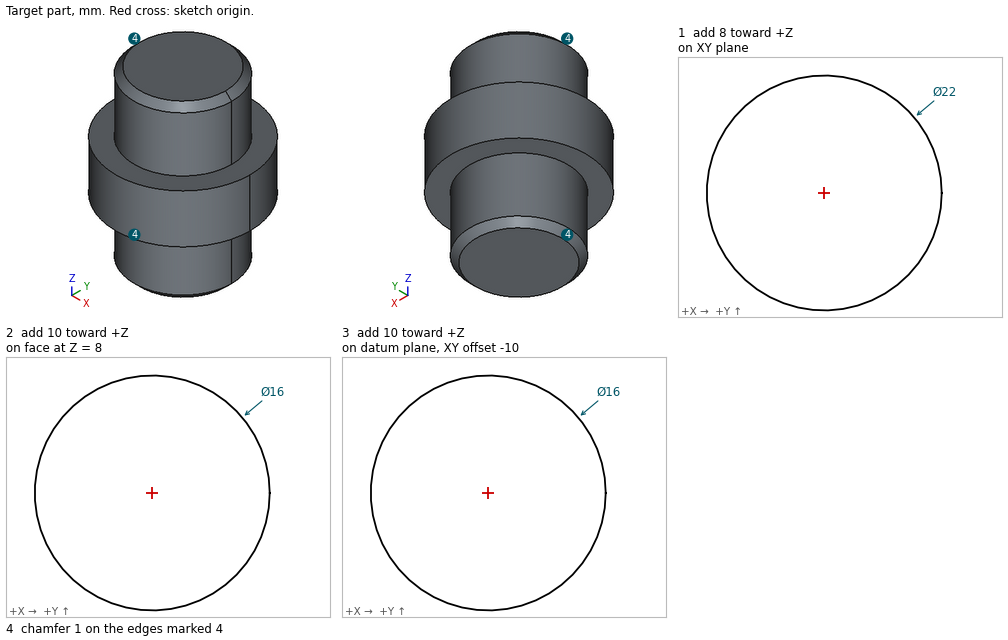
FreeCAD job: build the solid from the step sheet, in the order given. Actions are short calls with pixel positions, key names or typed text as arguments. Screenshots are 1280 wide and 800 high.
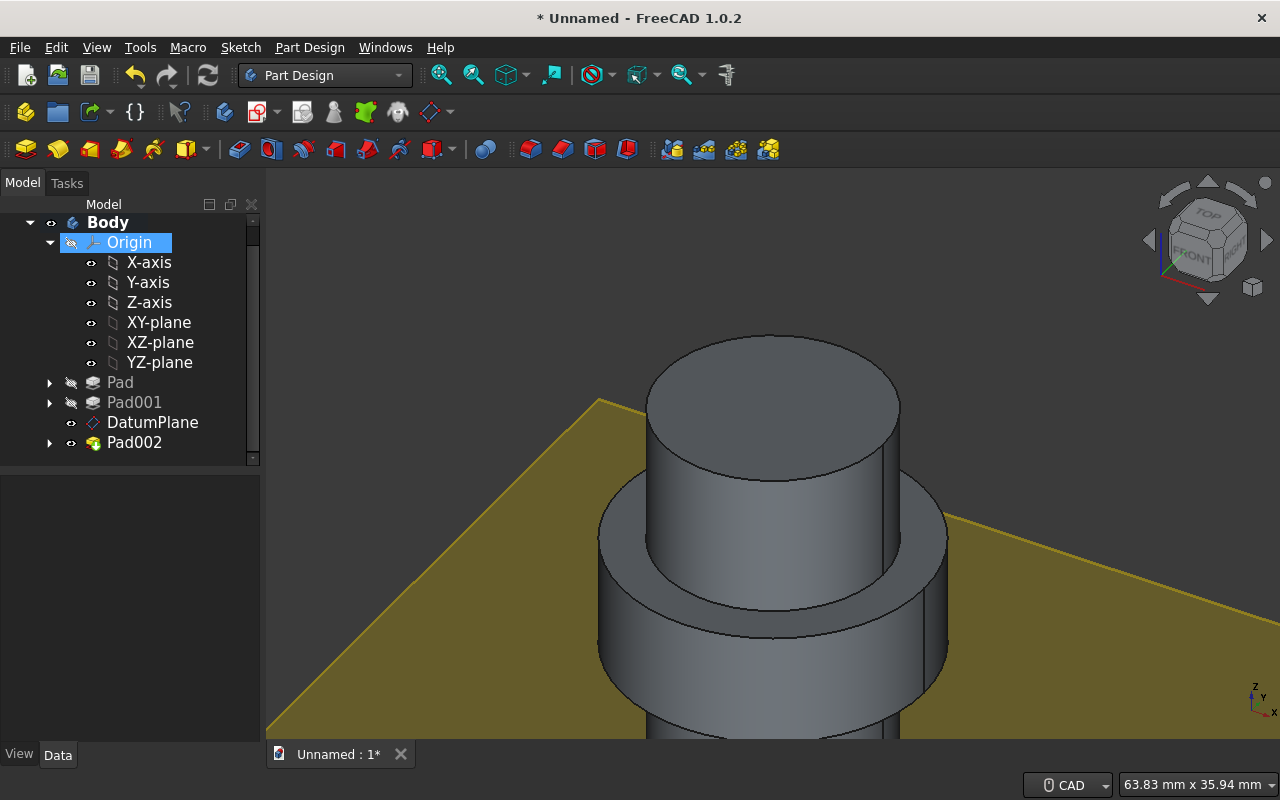
click(116, 423)
key(space)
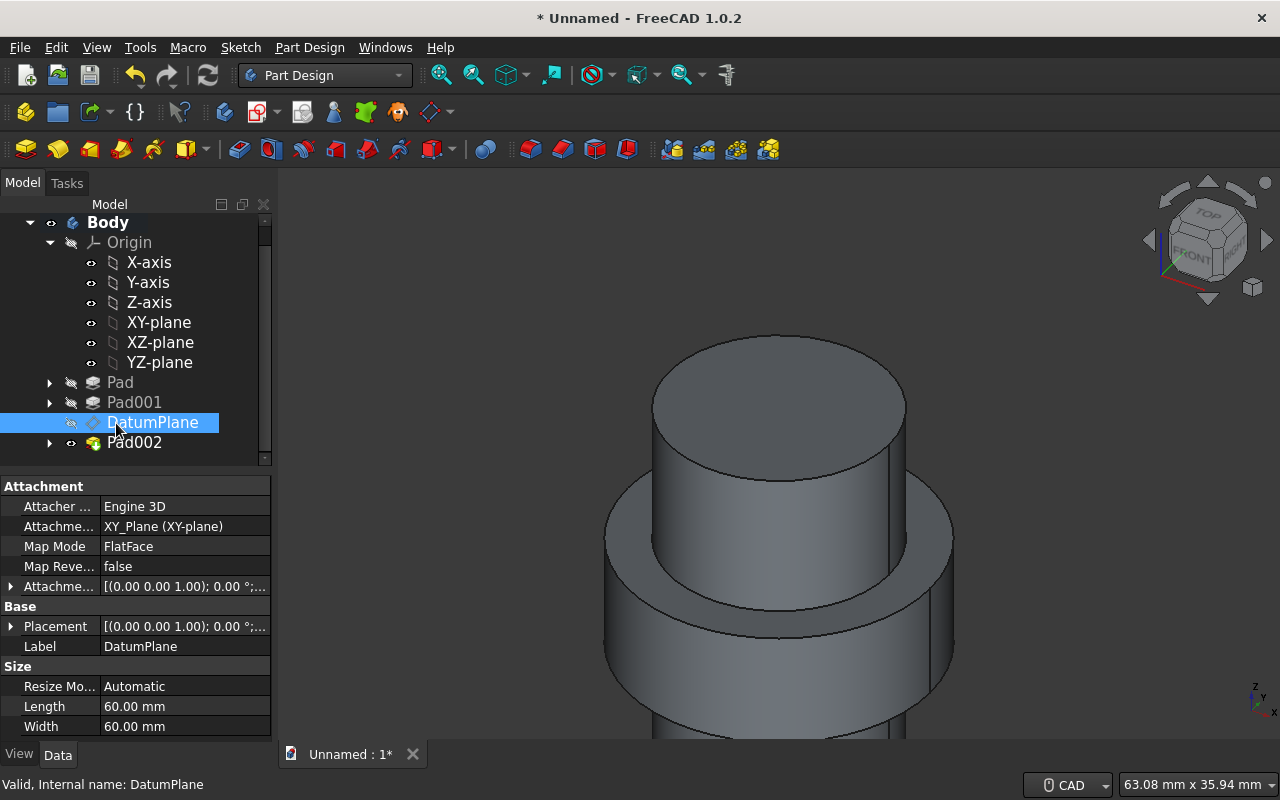
click(442, 76)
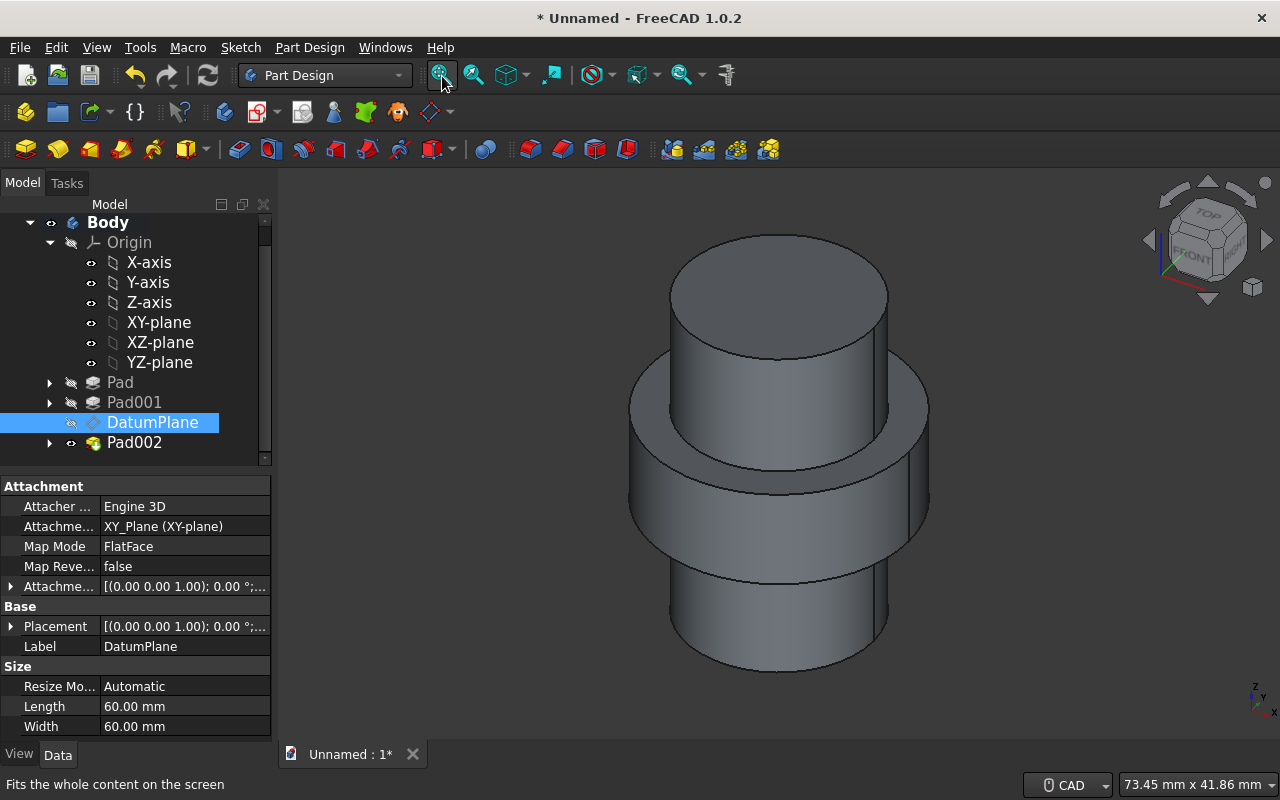
click(698, 651)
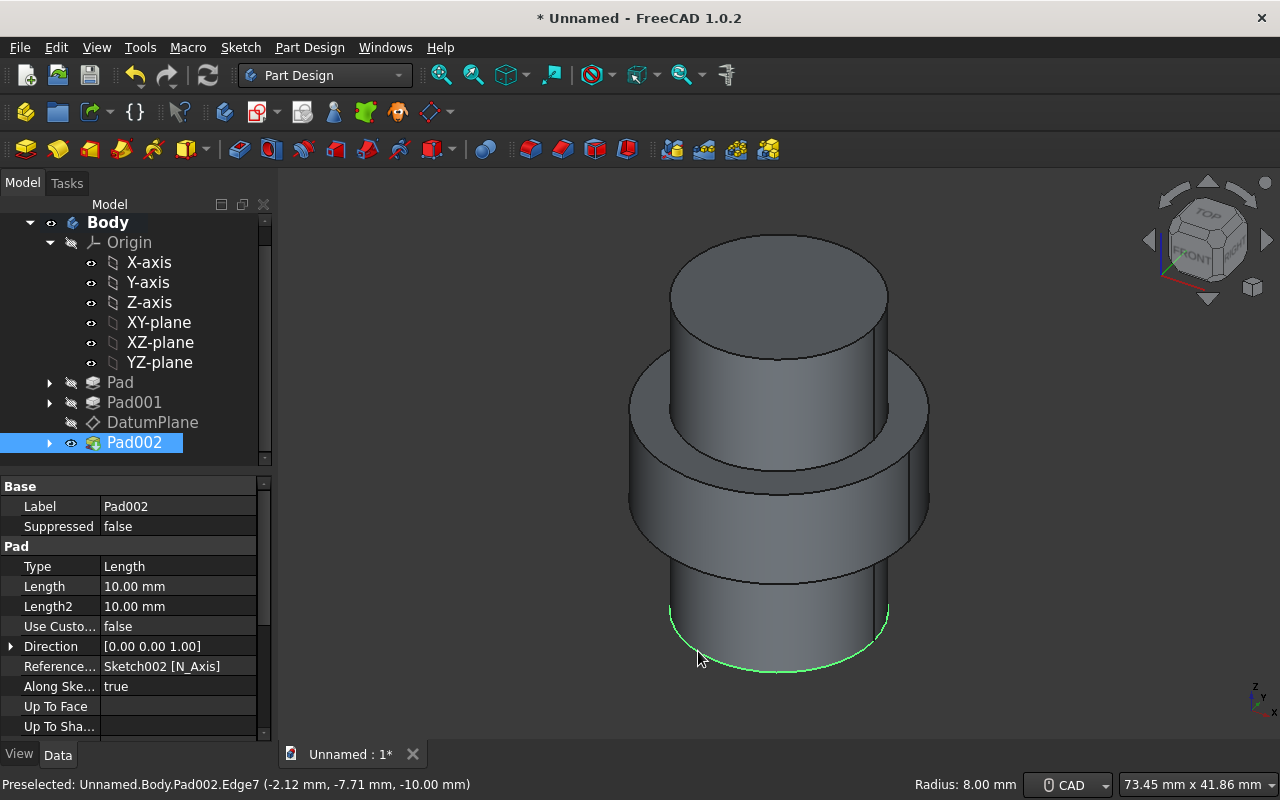
click(670, 303, ctrl)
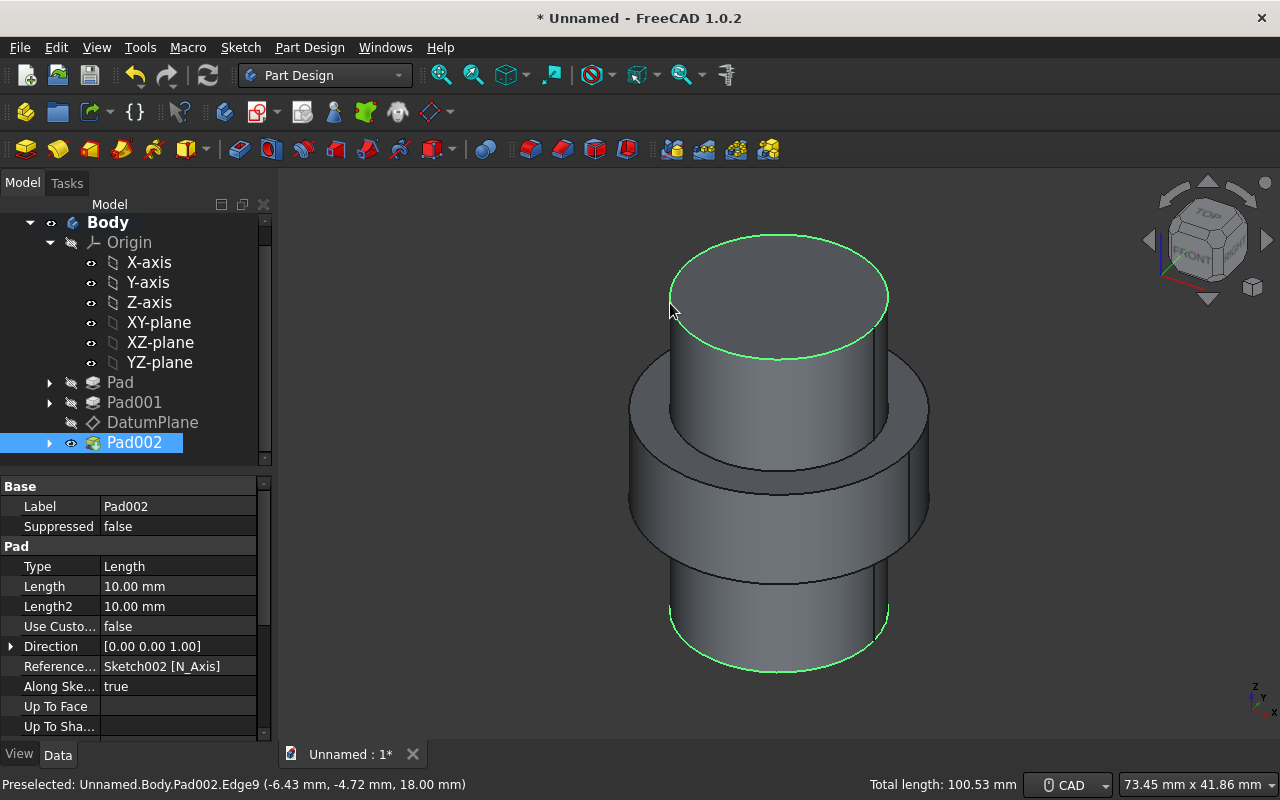
click(564, 150)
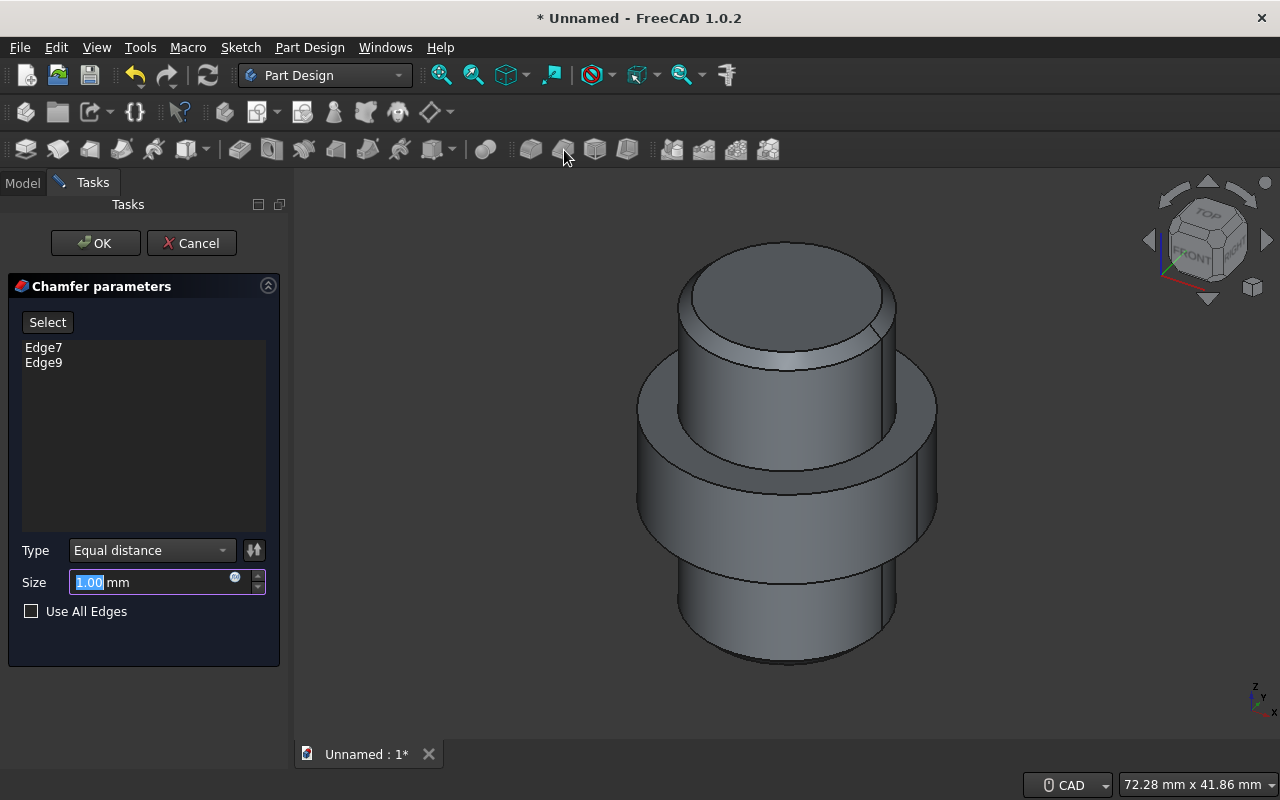
text(1)
key(Tab)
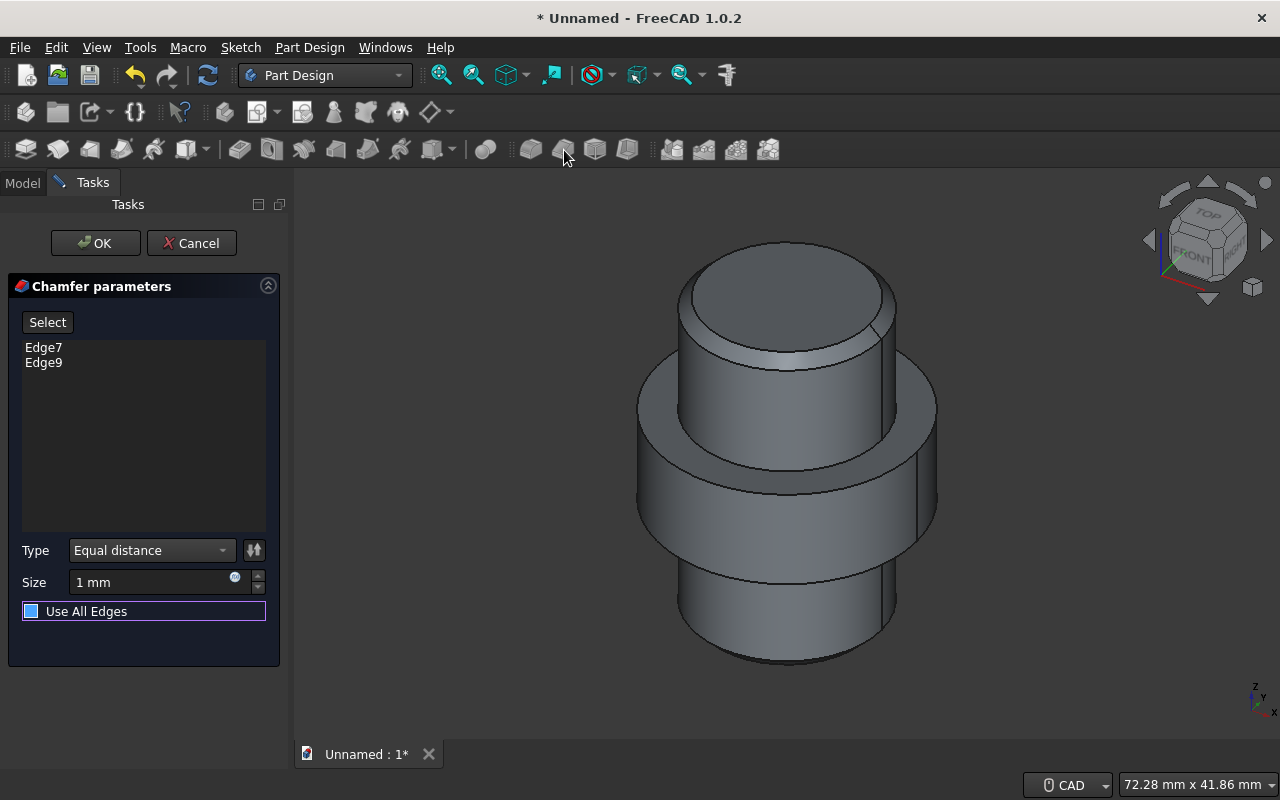
click(96, 243)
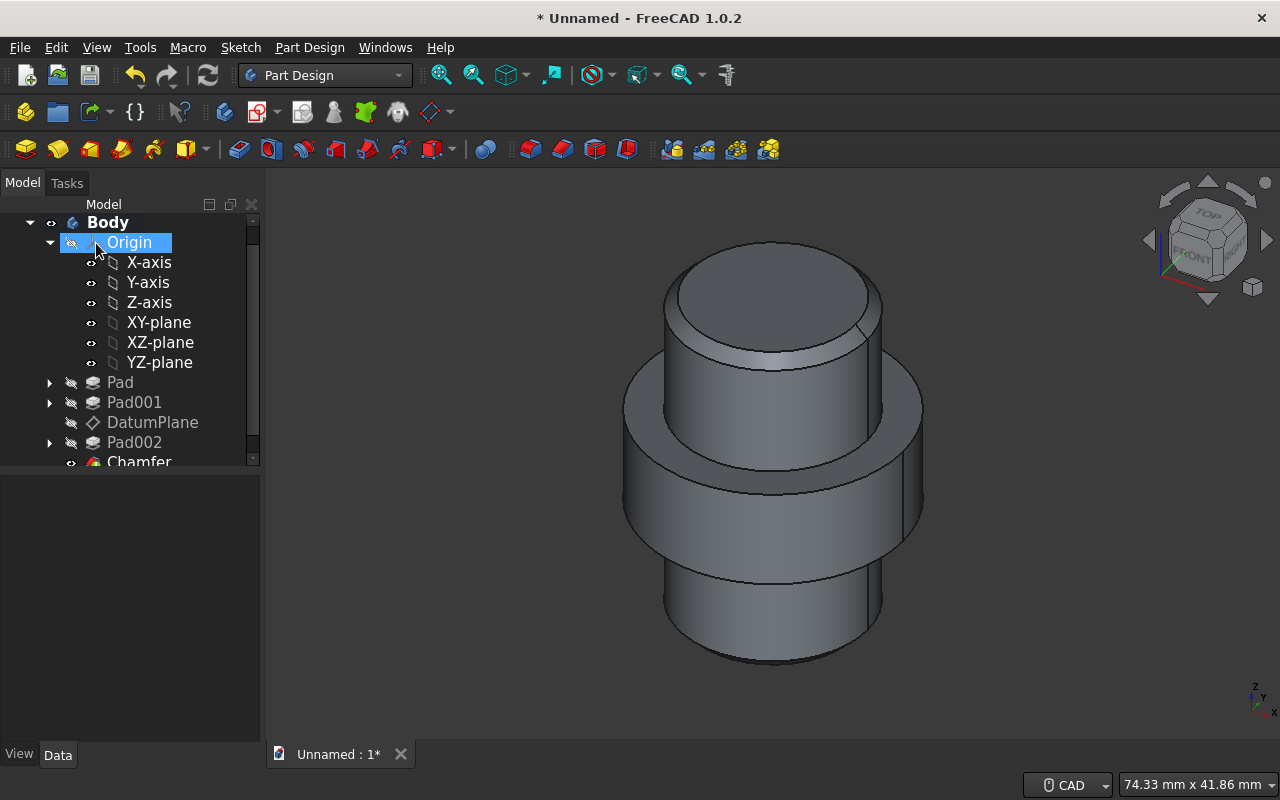
key(0)